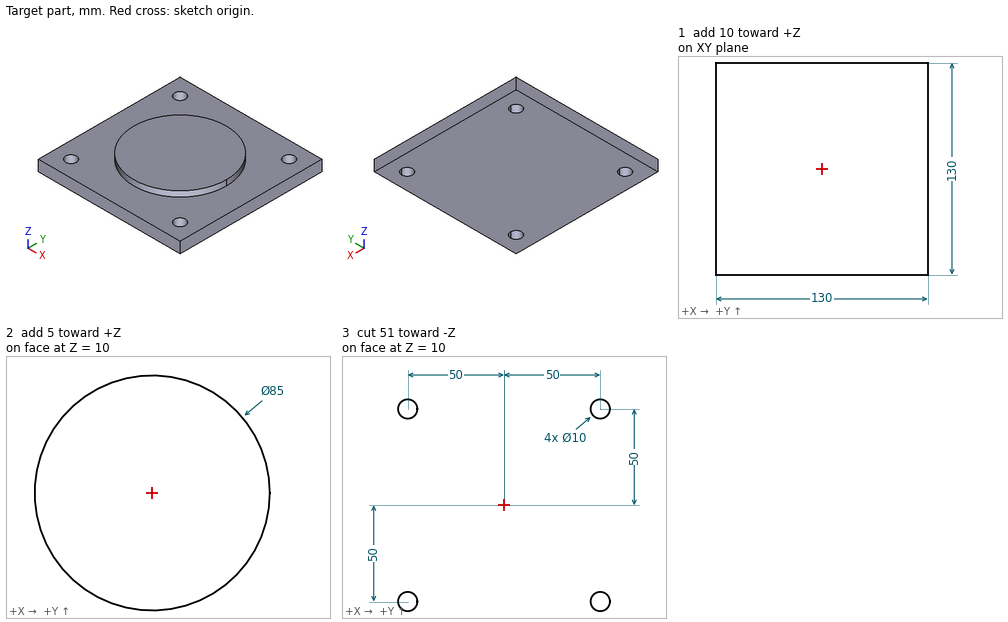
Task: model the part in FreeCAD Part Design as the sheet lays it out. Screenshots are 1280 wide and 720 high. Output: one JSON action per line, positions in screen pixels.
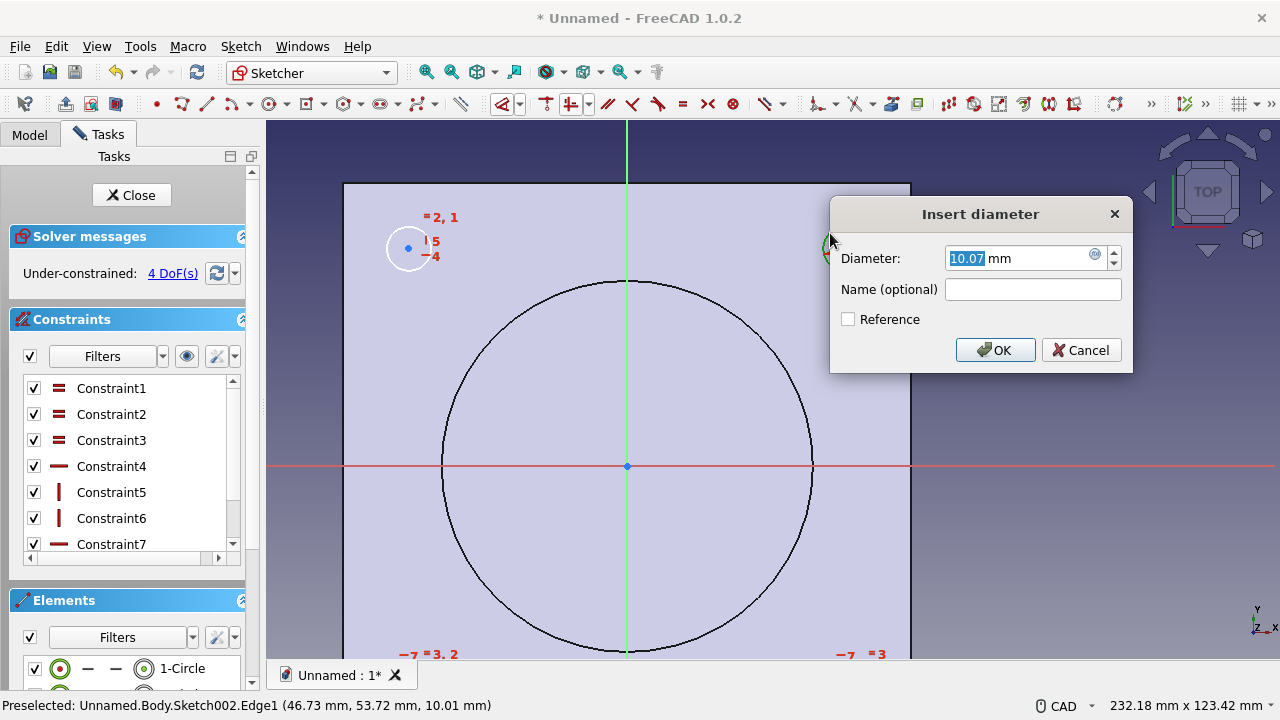
{"action": "type", "text": "10"}
{"action": "key", "text": "Return"}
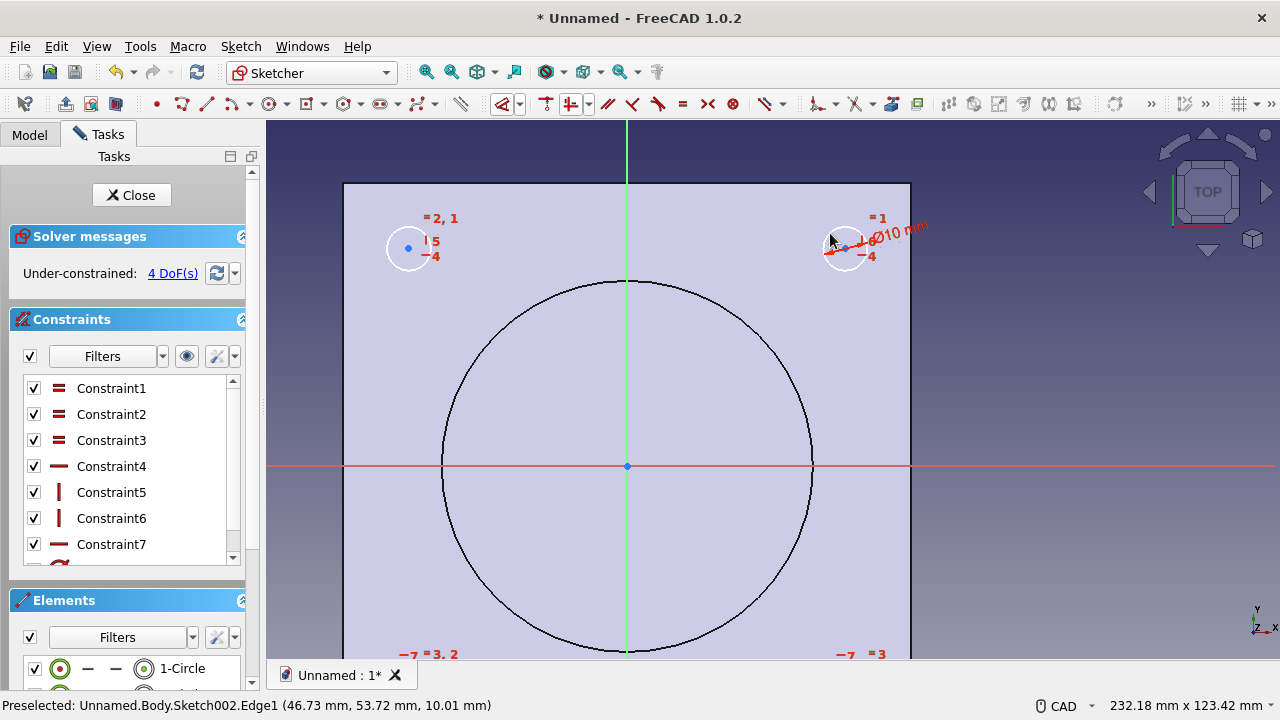
{"action": "left_click", "coordinate": [845, 249]}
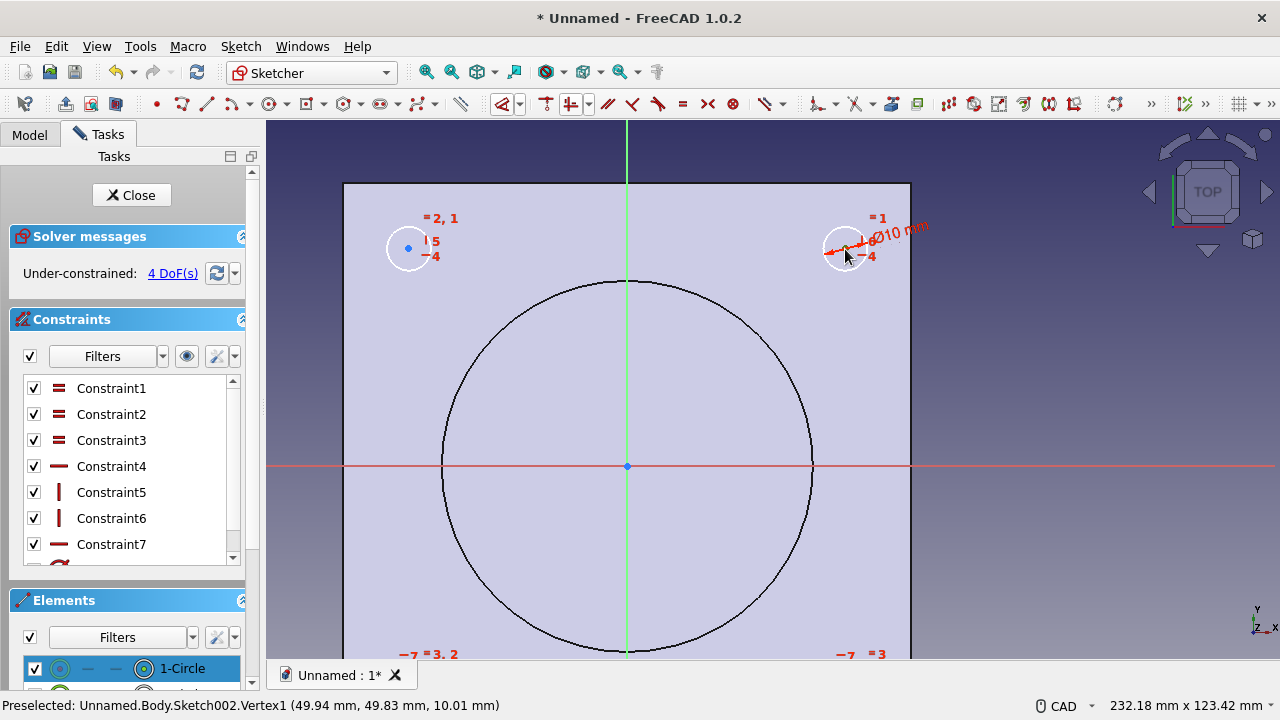
{"action": "left_click", "coordinate": [520, 104]}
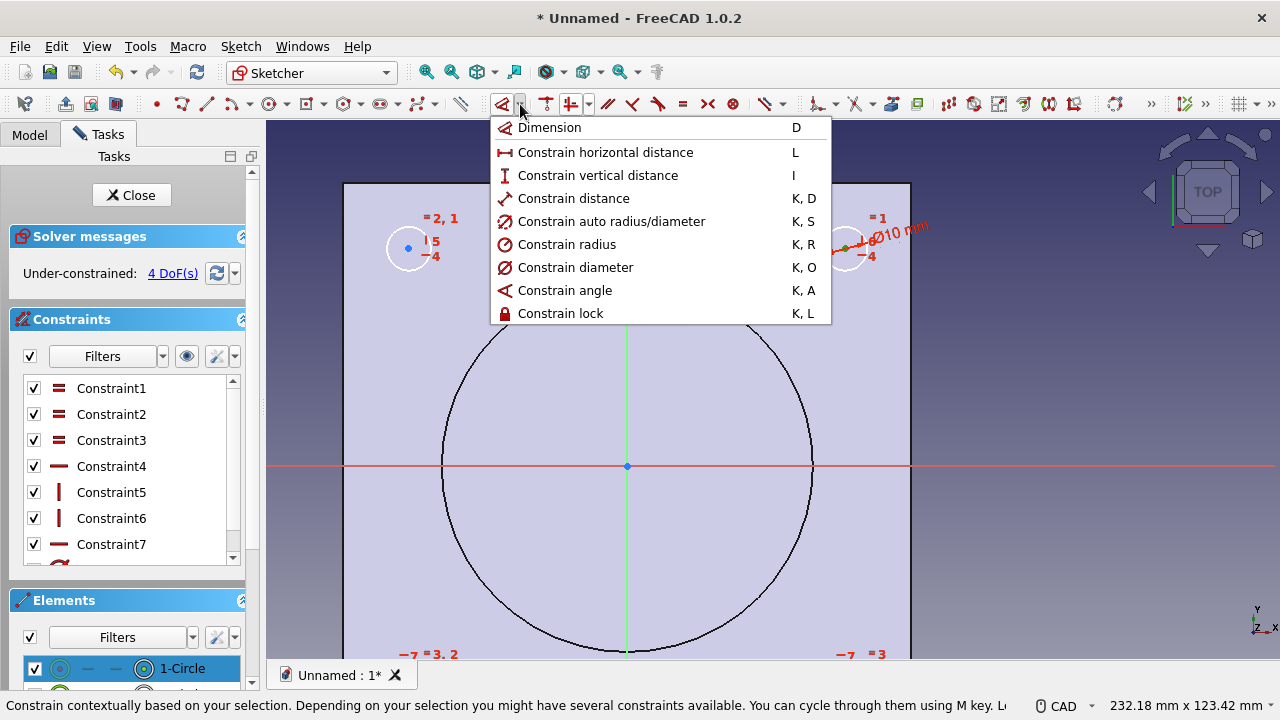
{"action": "left_click", "coordinate": [661, 152]}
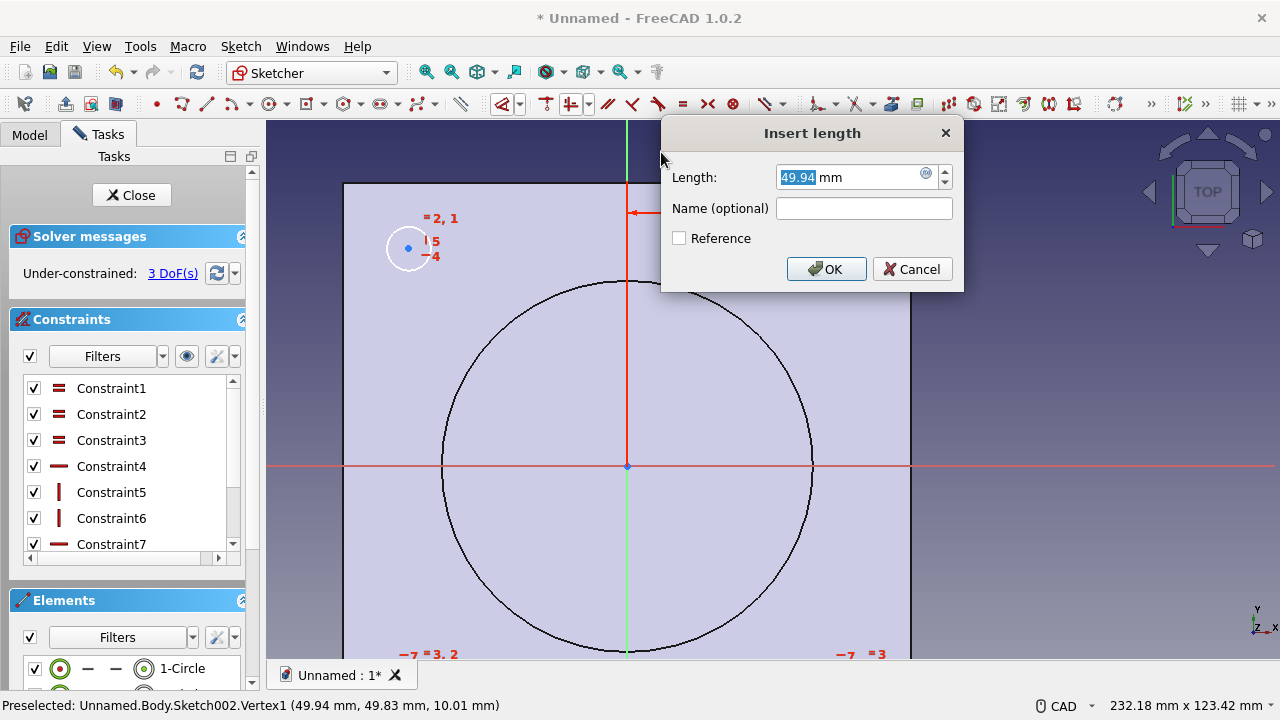
{"action": "type", "text": "50"}
{"action": "key", "text": "Return"}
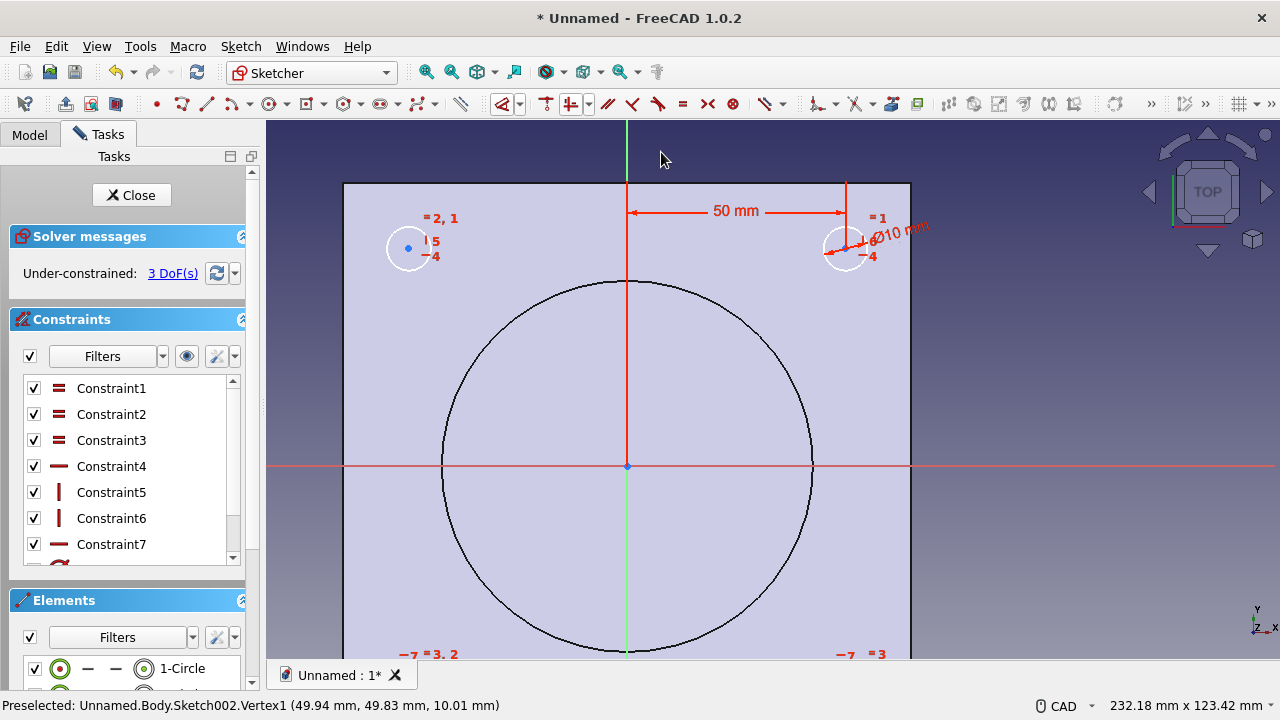
{"action": "left_click", "coordinate": [846, 249]}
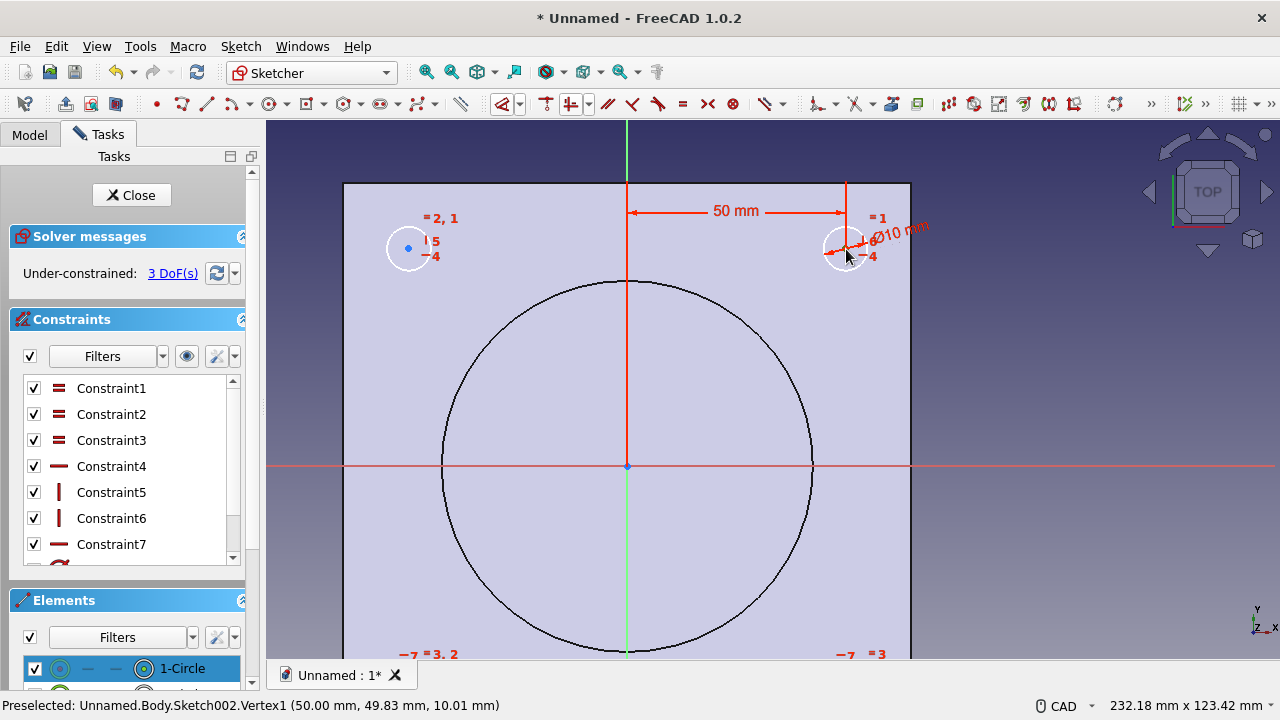
{"action": "key", "text": "i"}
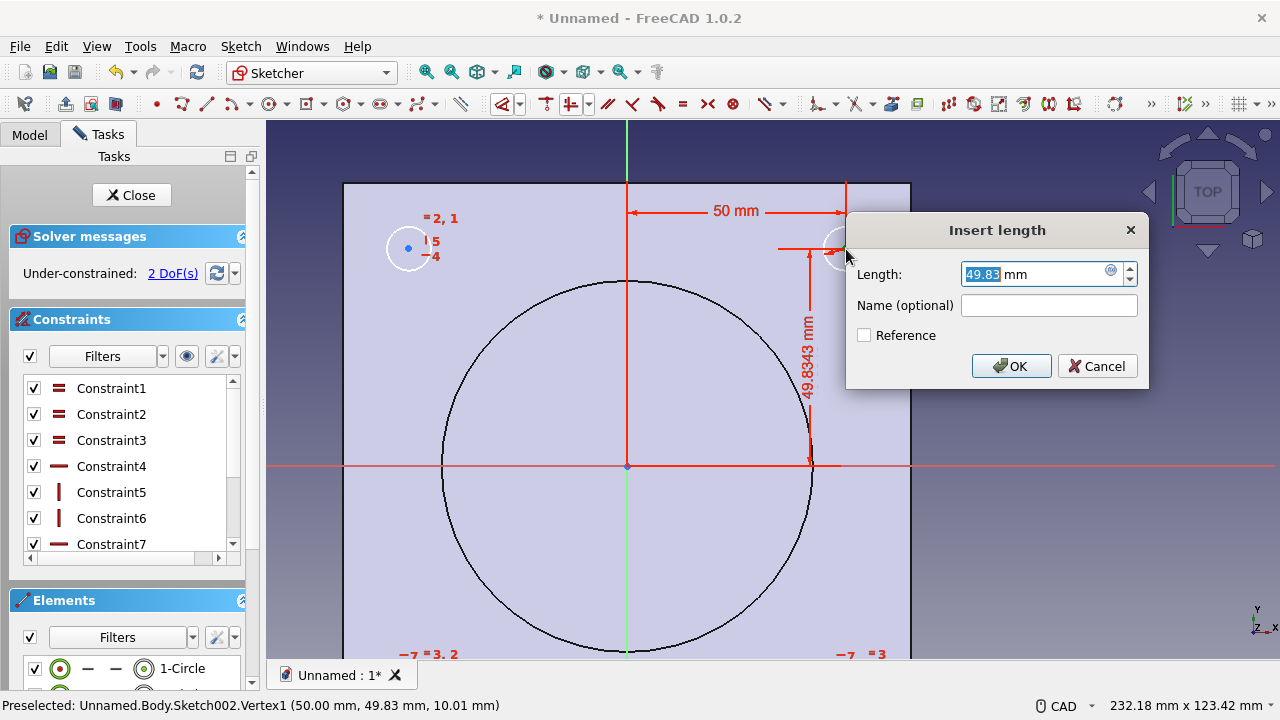
{"action": "type", "text": "50"}
{"action": "key", "text": "Return"}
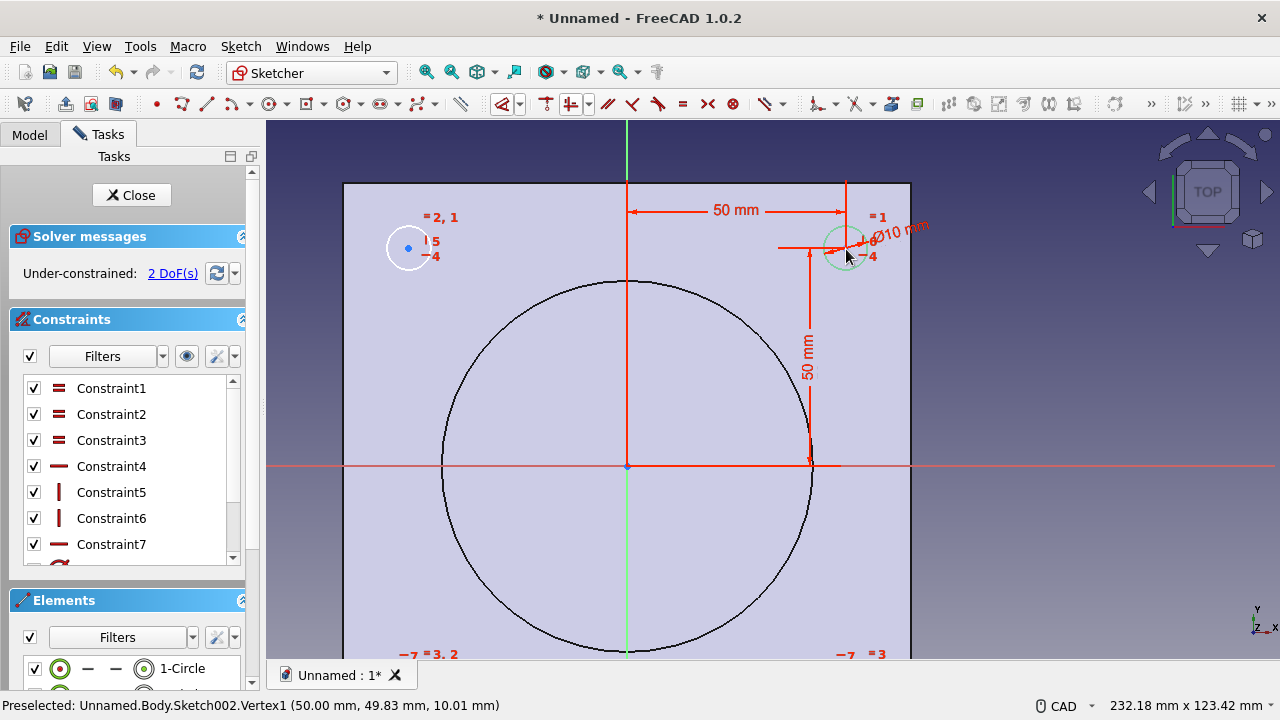
{"action": "left_click", "coordinate": [409, 248]}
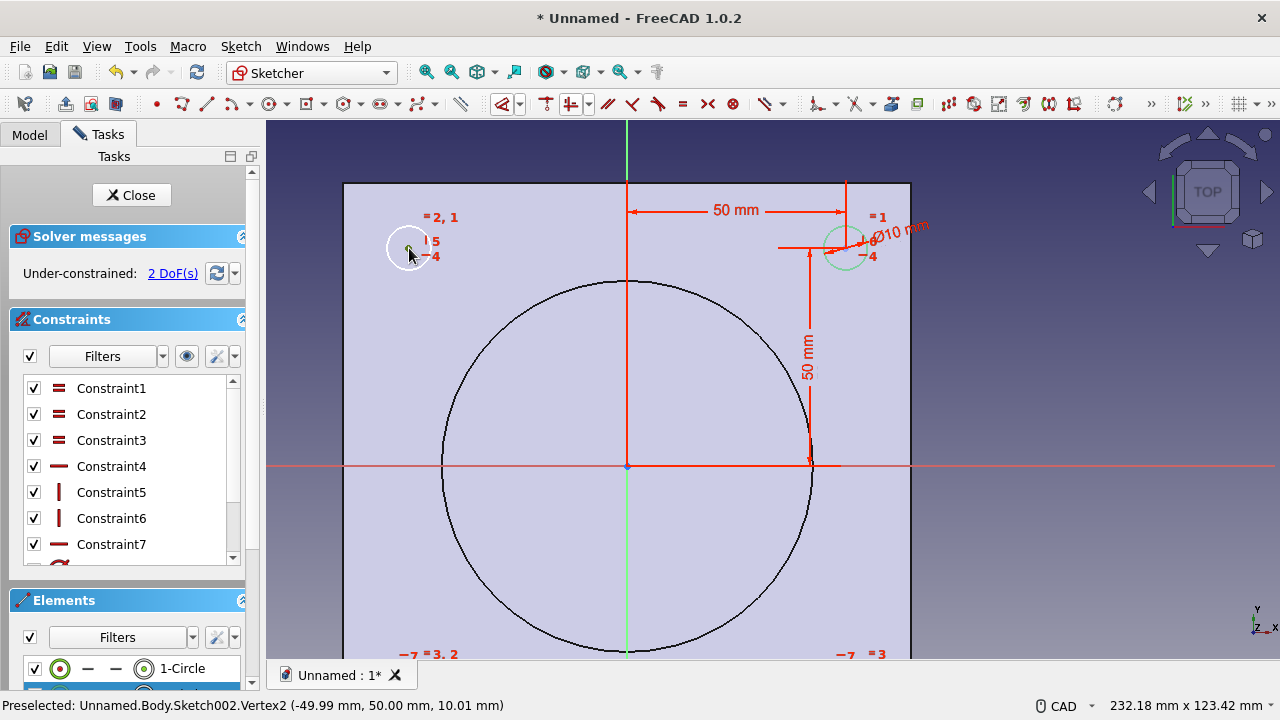
{"action": "key", "text": "l"}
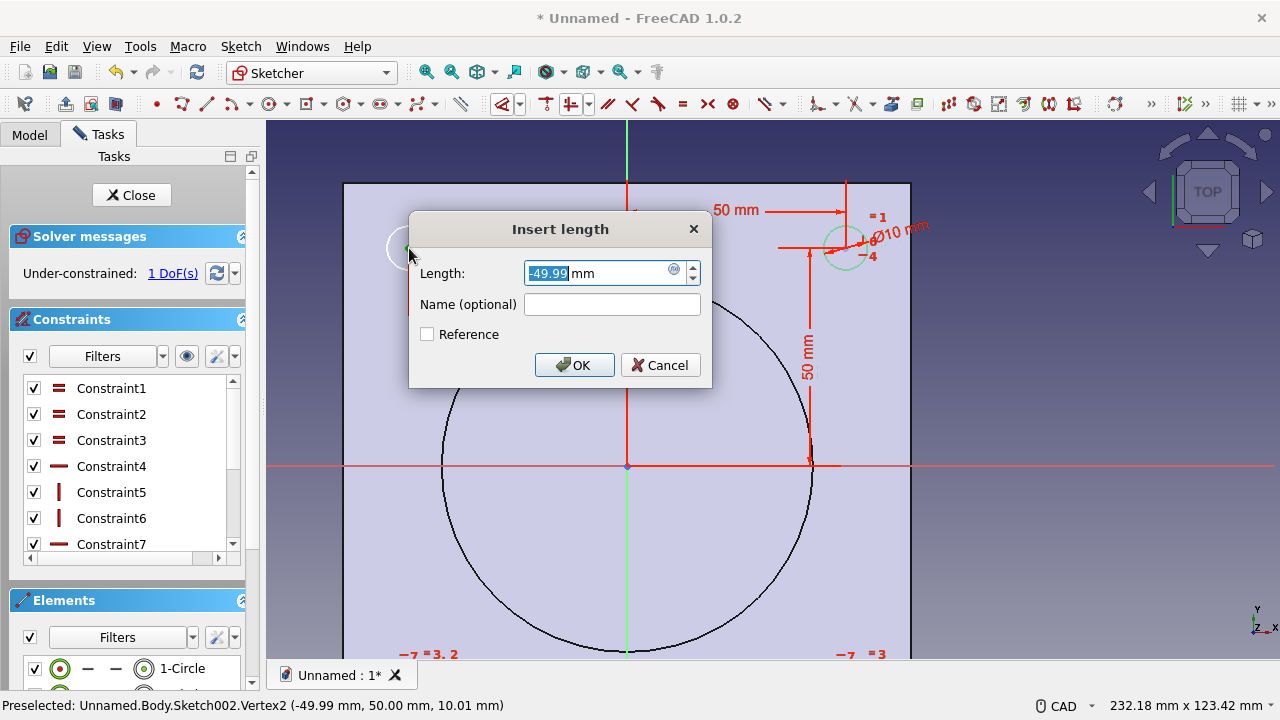
{"action": "type", "text": "-50"}
{"action": "key", "text": "Return"}